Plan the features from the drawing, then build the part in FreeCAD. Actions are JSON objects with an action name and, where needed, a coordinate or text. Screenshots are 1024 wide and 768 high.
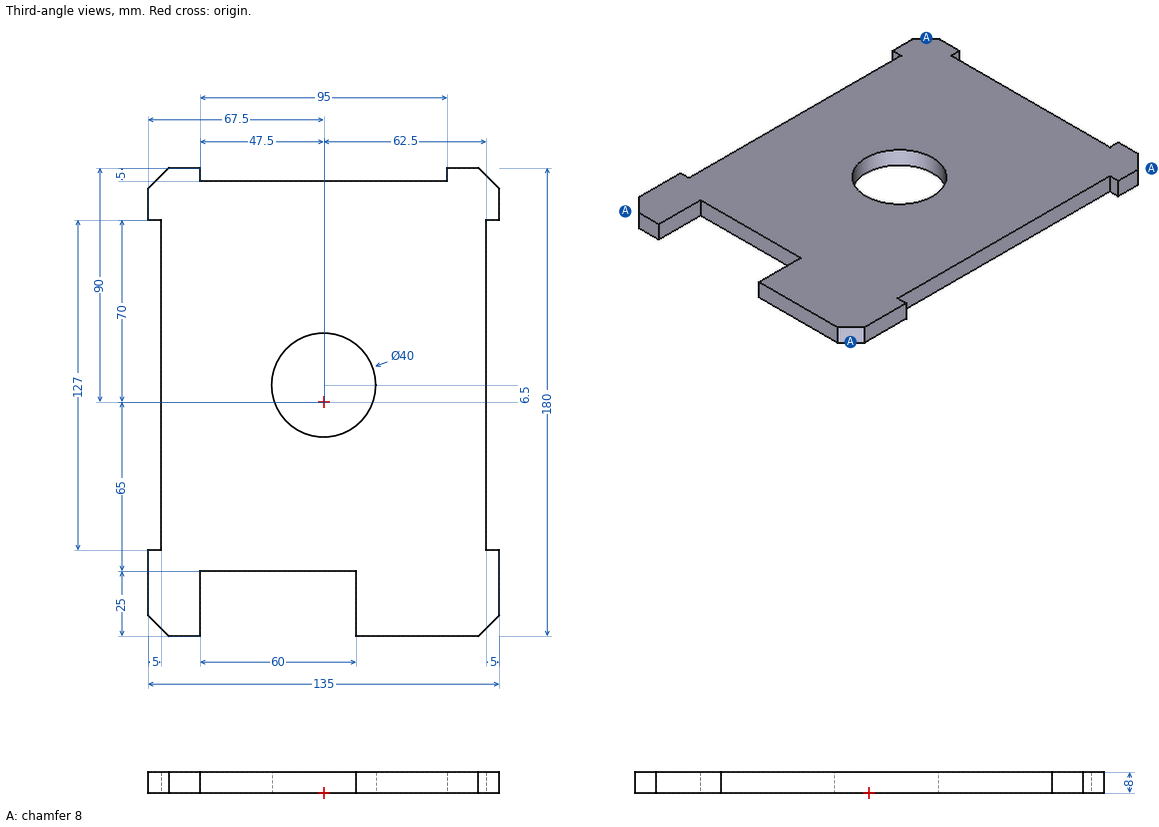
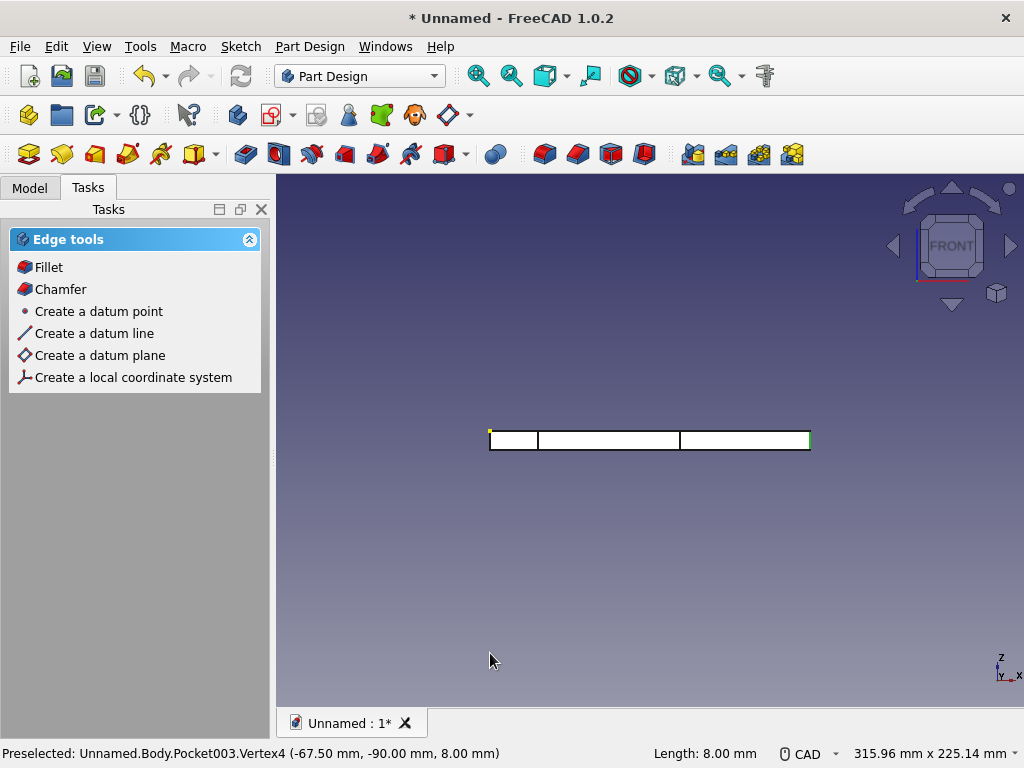
{"action": "key", "text": "v f"}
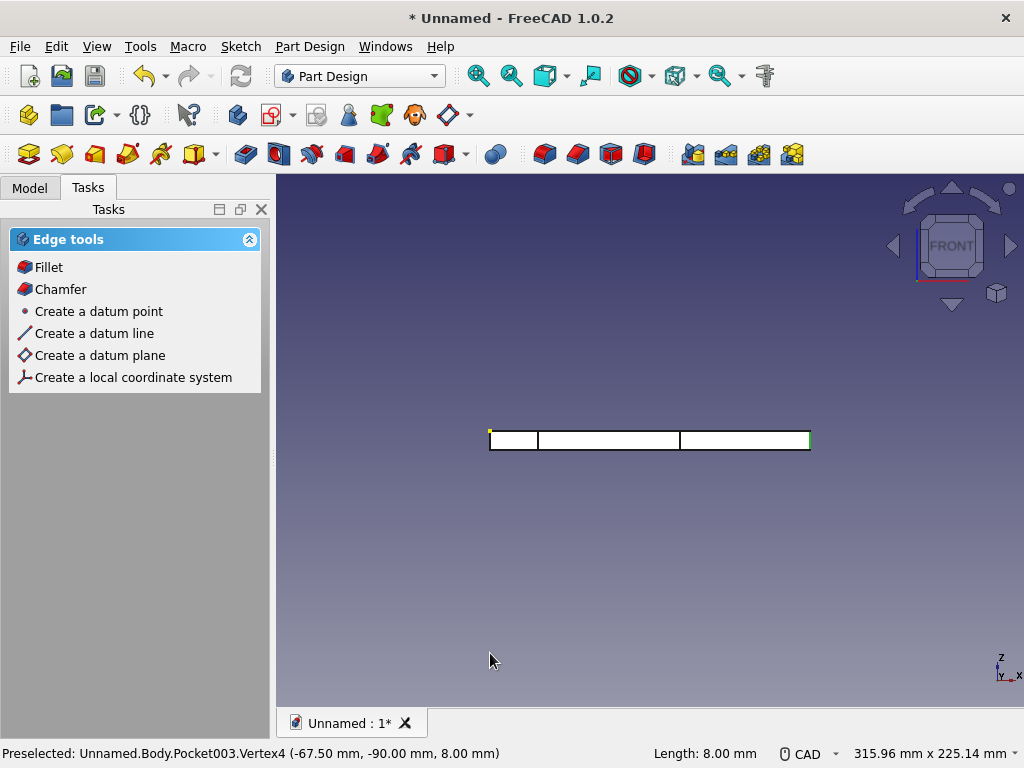
{"action": "left_click", "coordinate": [490, 440], "text": "ctrl"}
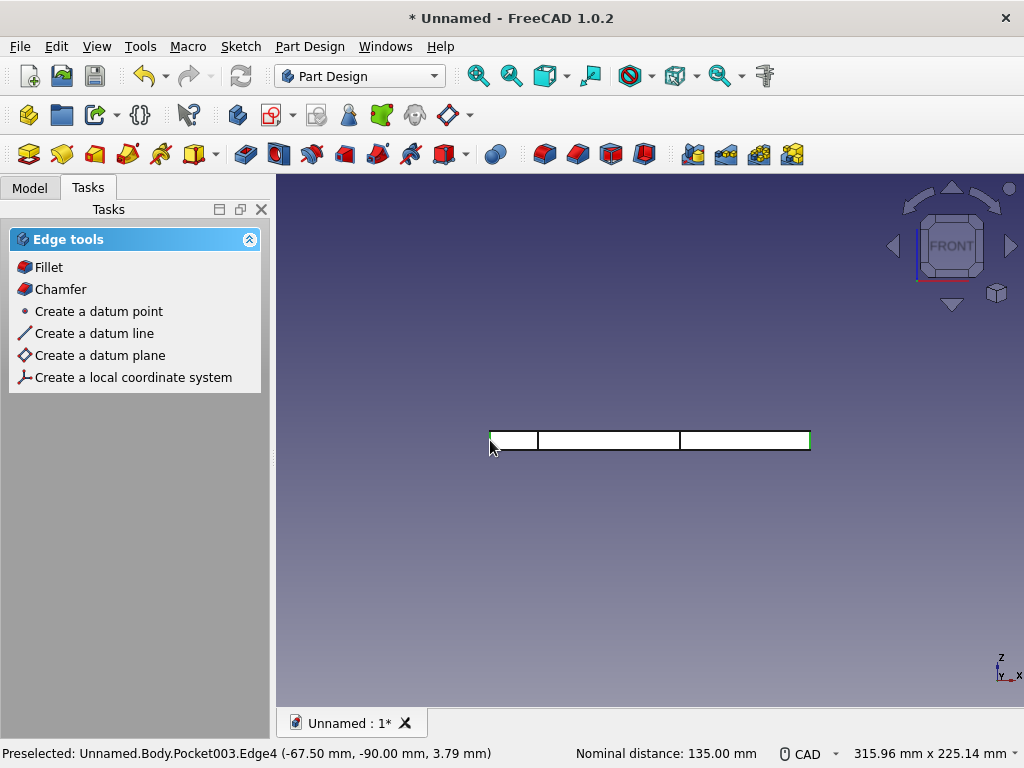
{"action": "scroll", "coordinate": [490, 440], "scroll_direction": "up", "scroll_amount": 4}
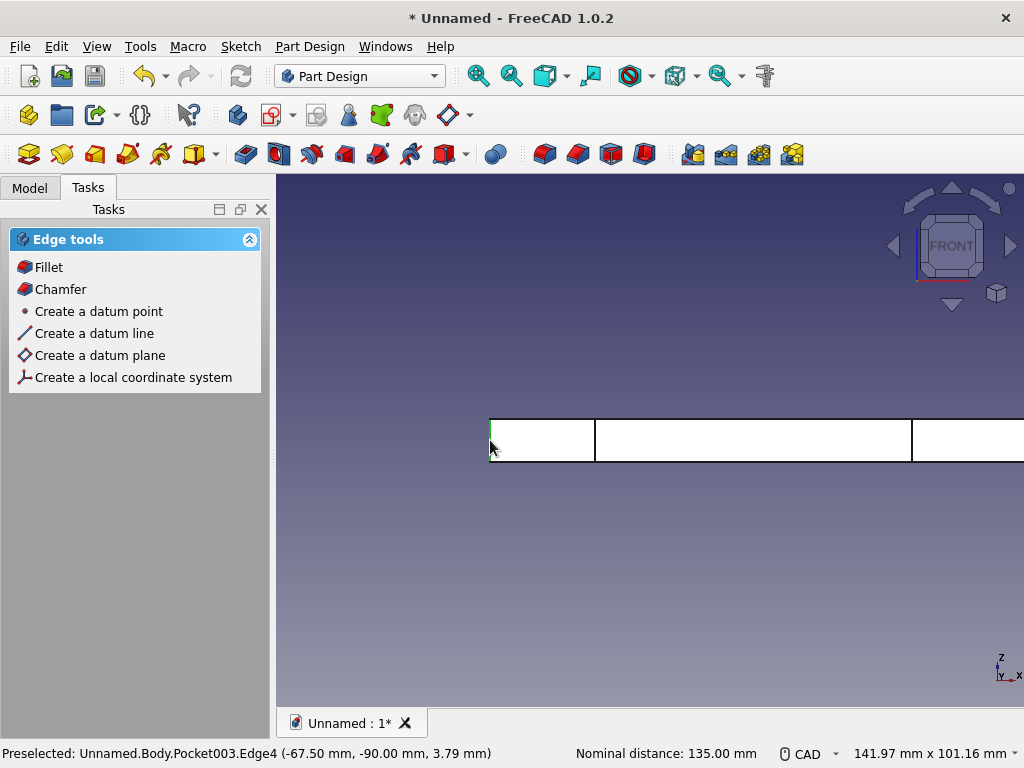
{"action": "key", "text": "v f"}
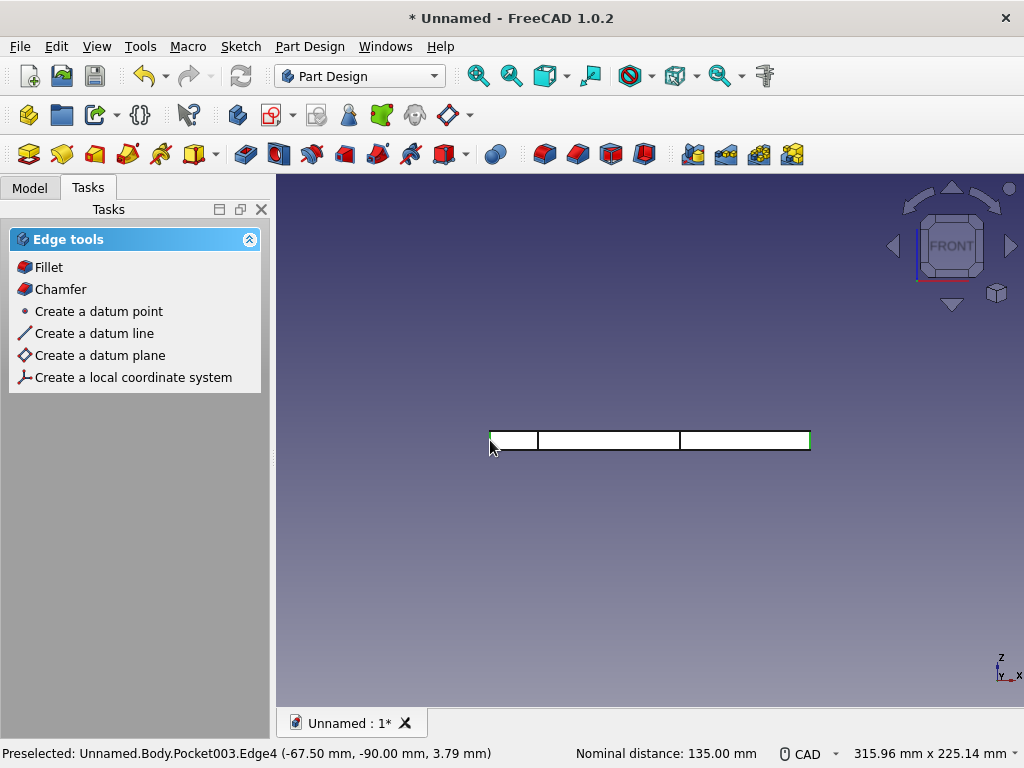
{"action": "key", "text": "3"}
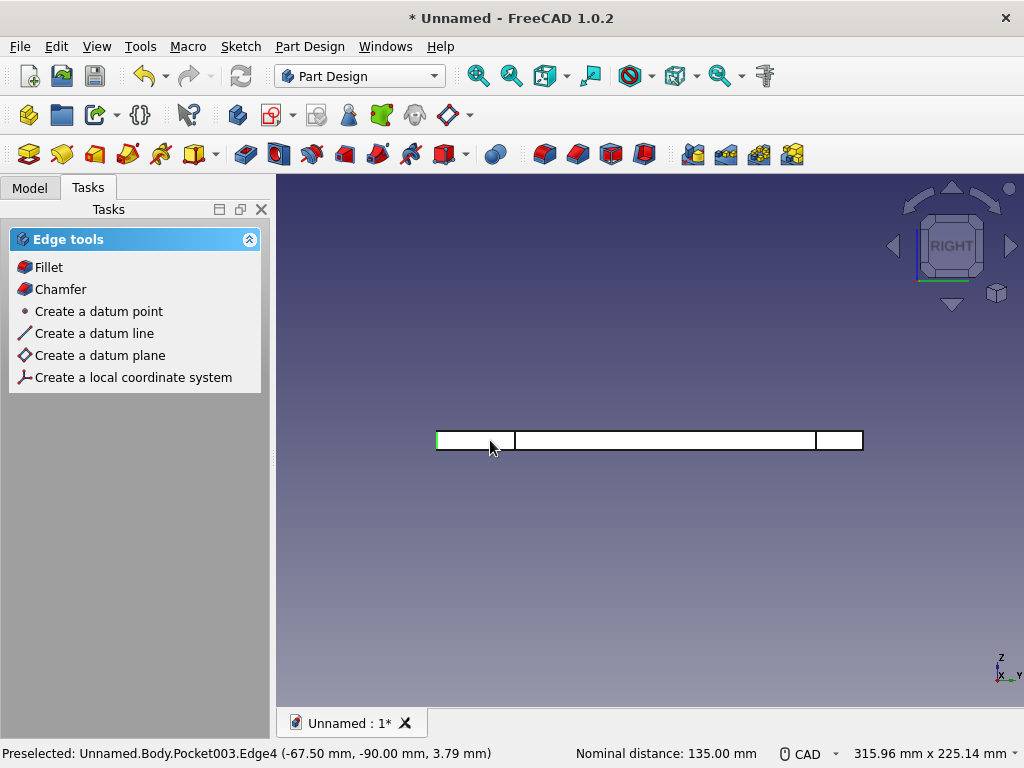
{"action": "left_click", "coordinate": [863, 439], "text": "ctrl"}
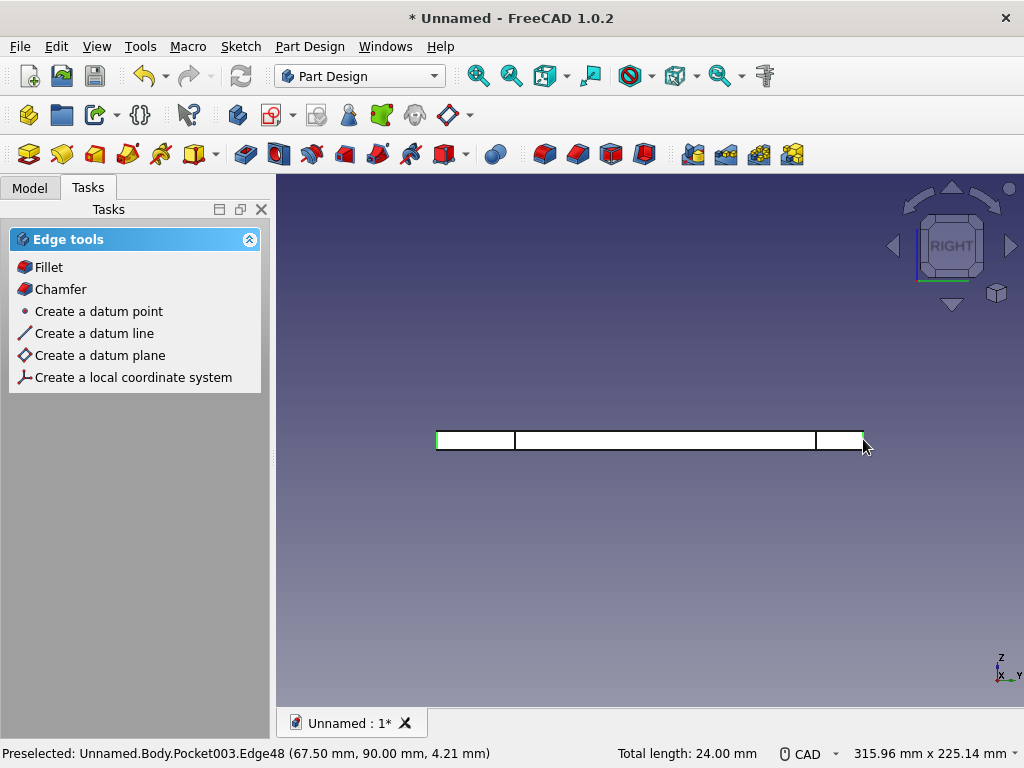
{"action": "key", "text": "5"}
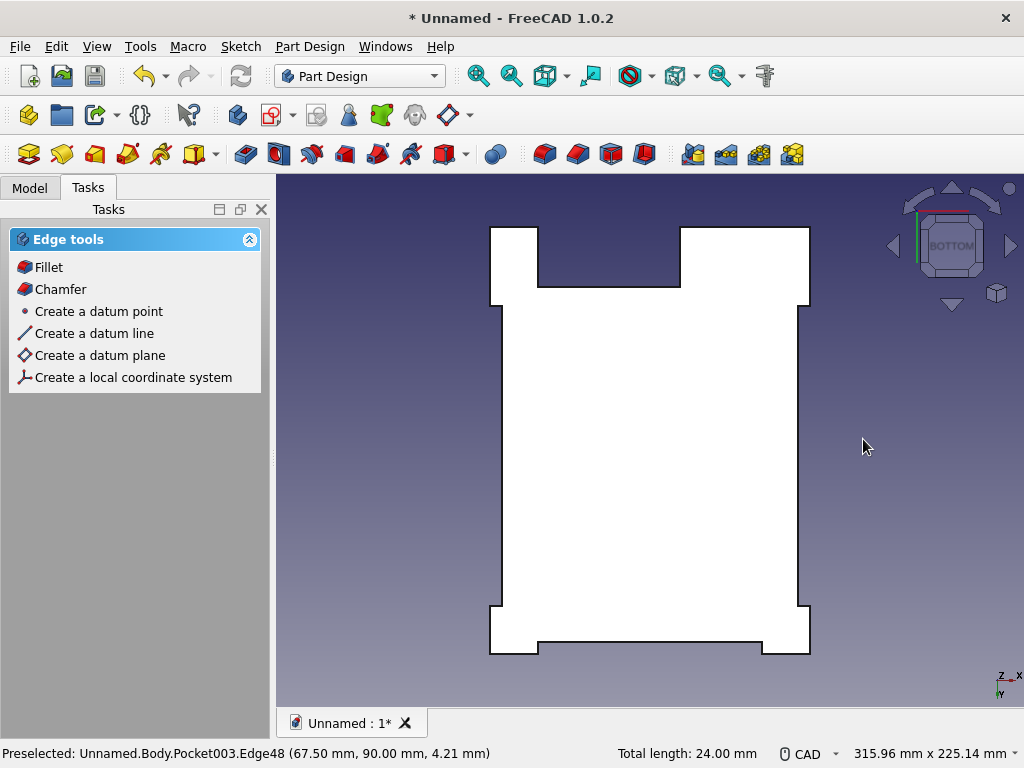
{"action": "scroll", "coordinate": [490, 653], "scroll_direction": "up", "scroll_amount": 4}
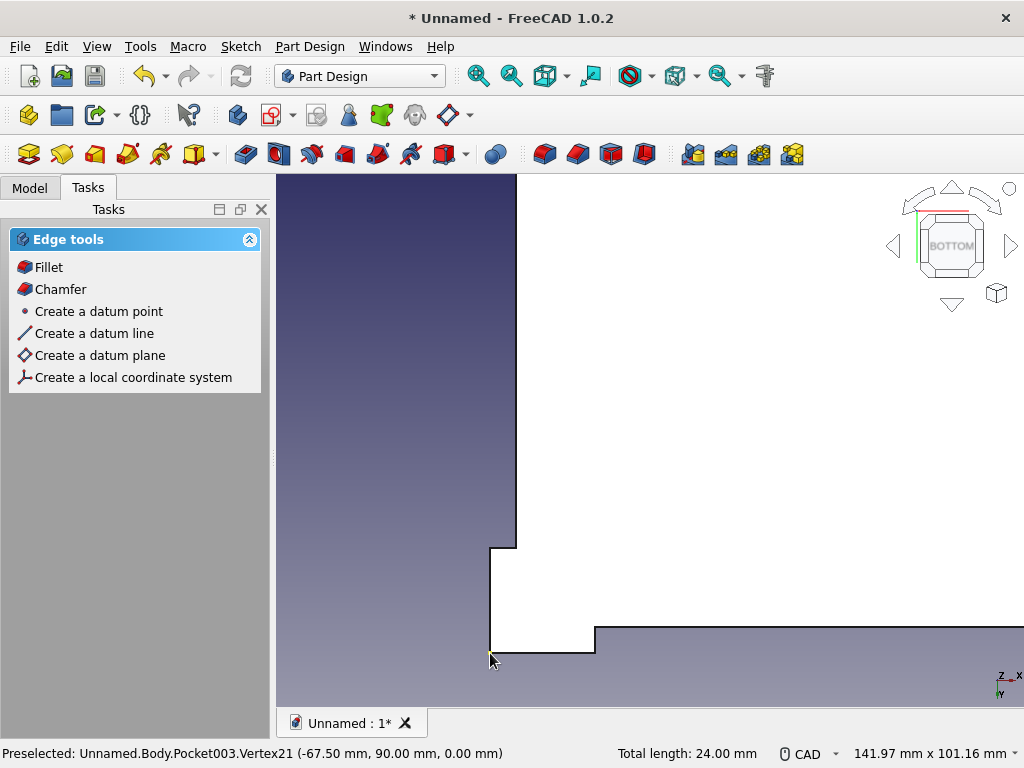
{"action": "key", "text": "v f"}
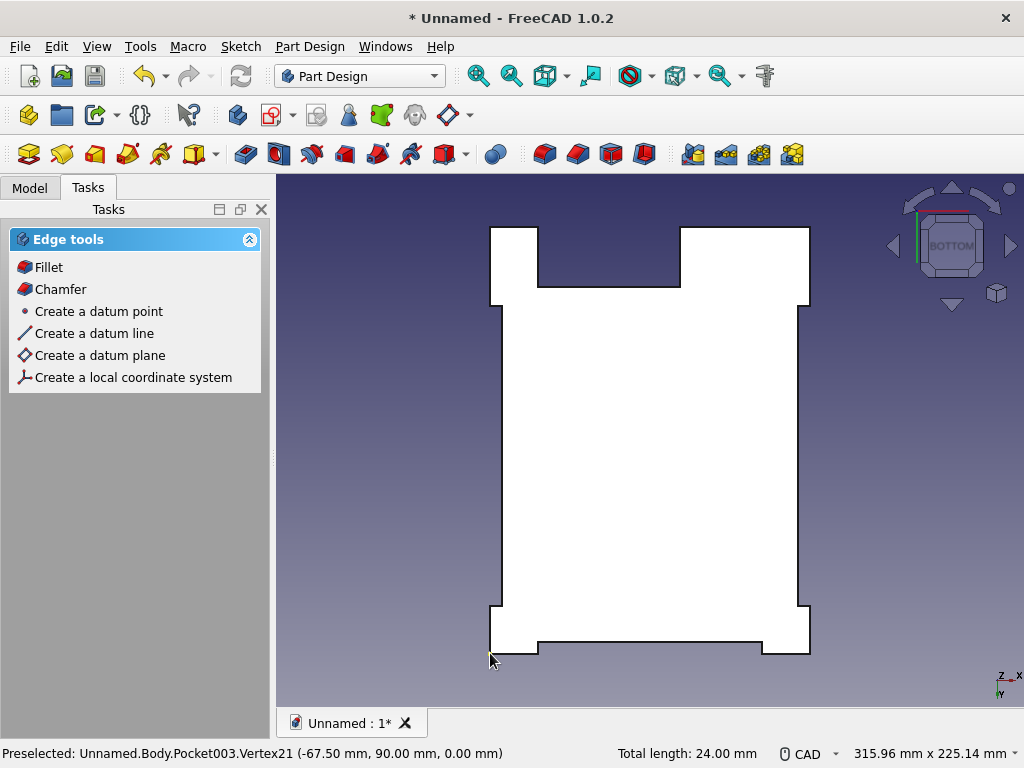
{"action": "key", "text": "4"}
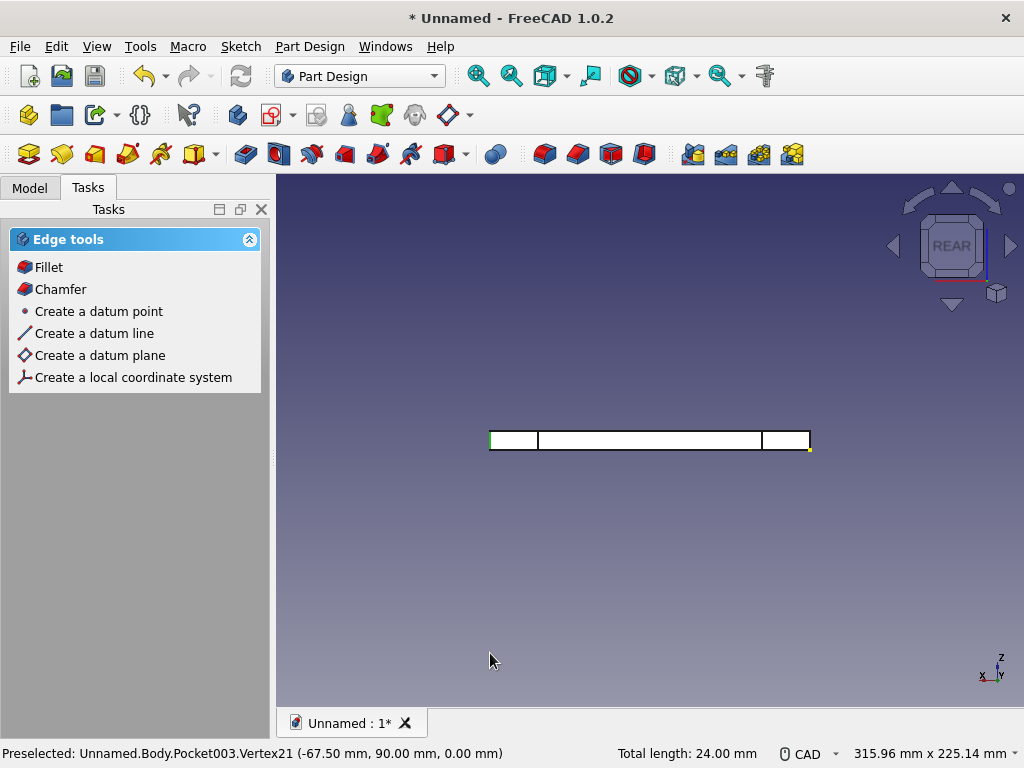
{"action": "key", "text": "v f"}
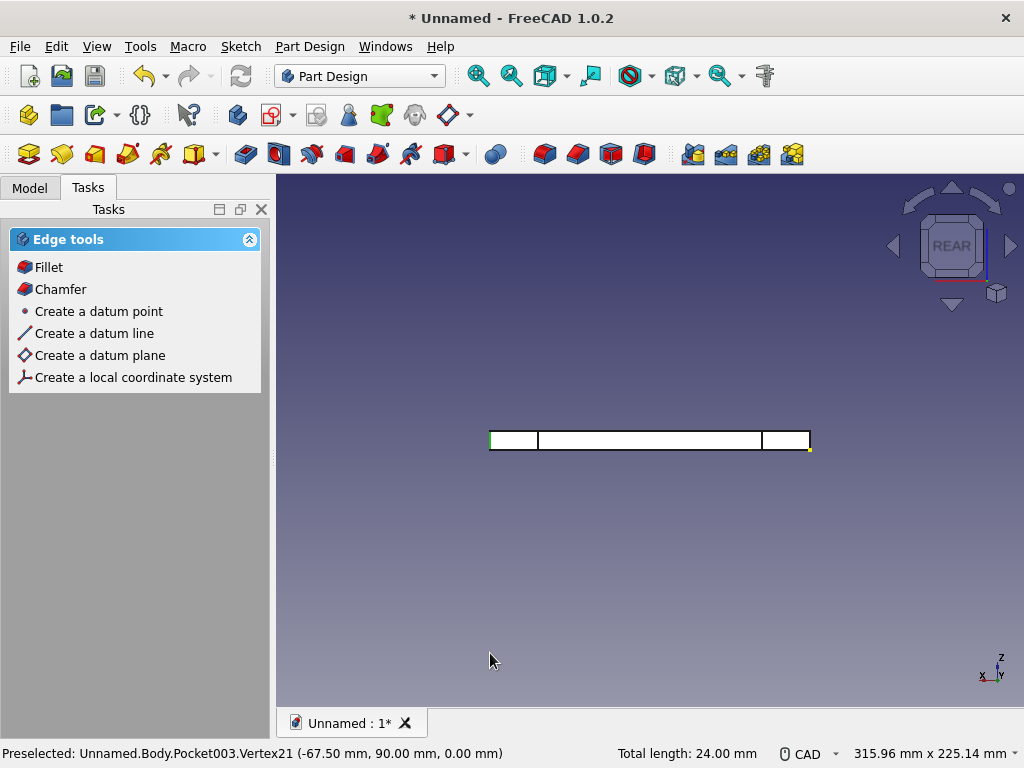
{"action": "left_click", "coordinate": [810, 440], "text": "ctrl"}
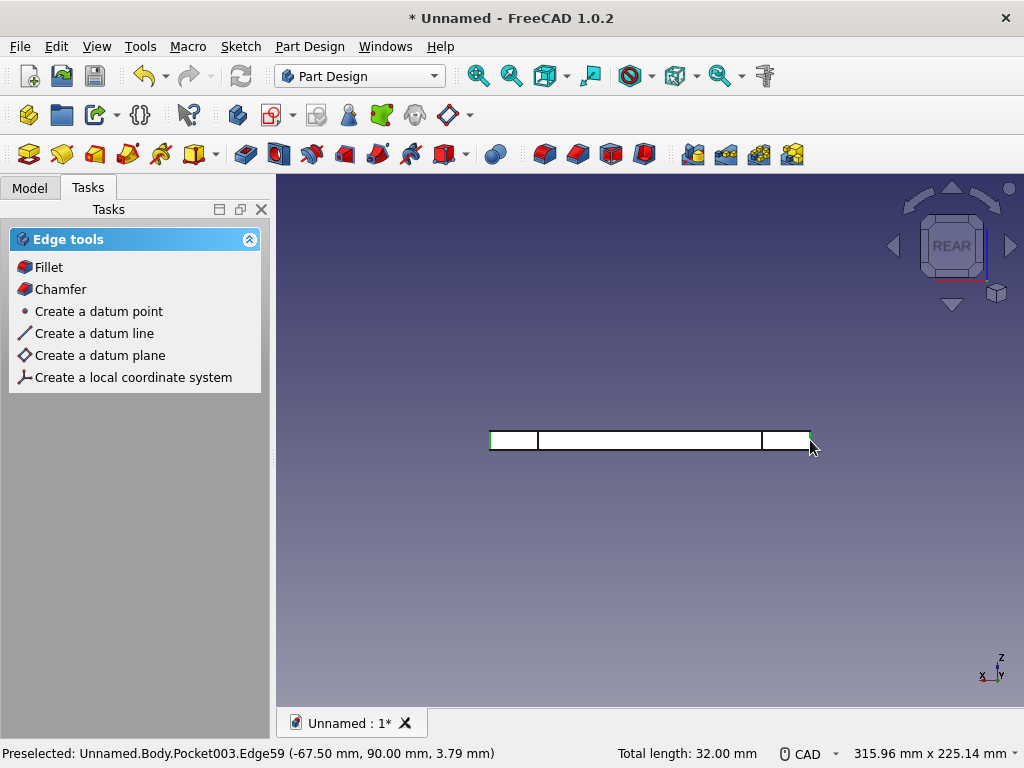
{"action": "left_click", "coordinate": [578, 154]}